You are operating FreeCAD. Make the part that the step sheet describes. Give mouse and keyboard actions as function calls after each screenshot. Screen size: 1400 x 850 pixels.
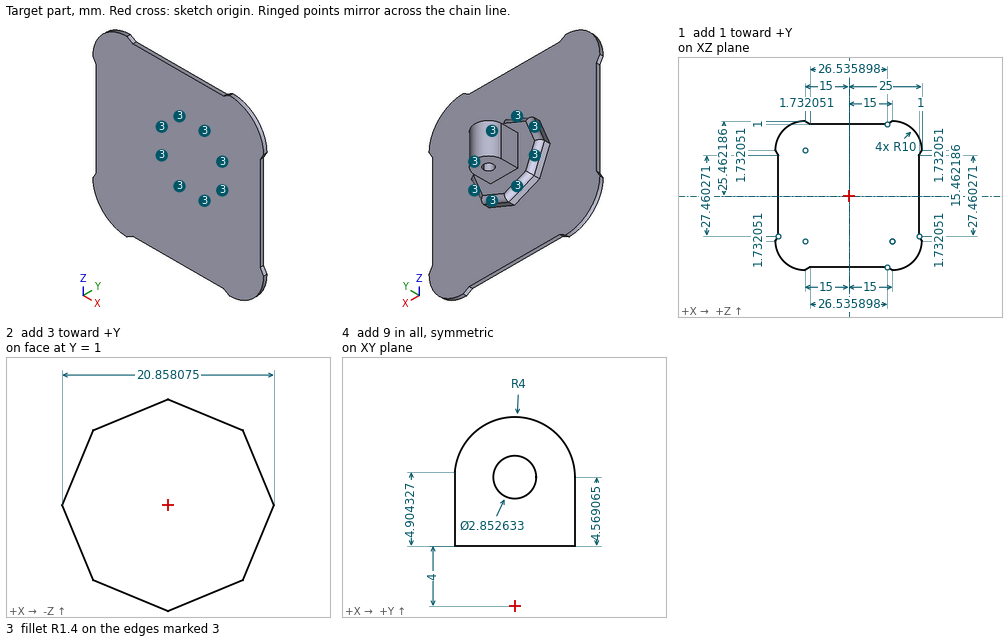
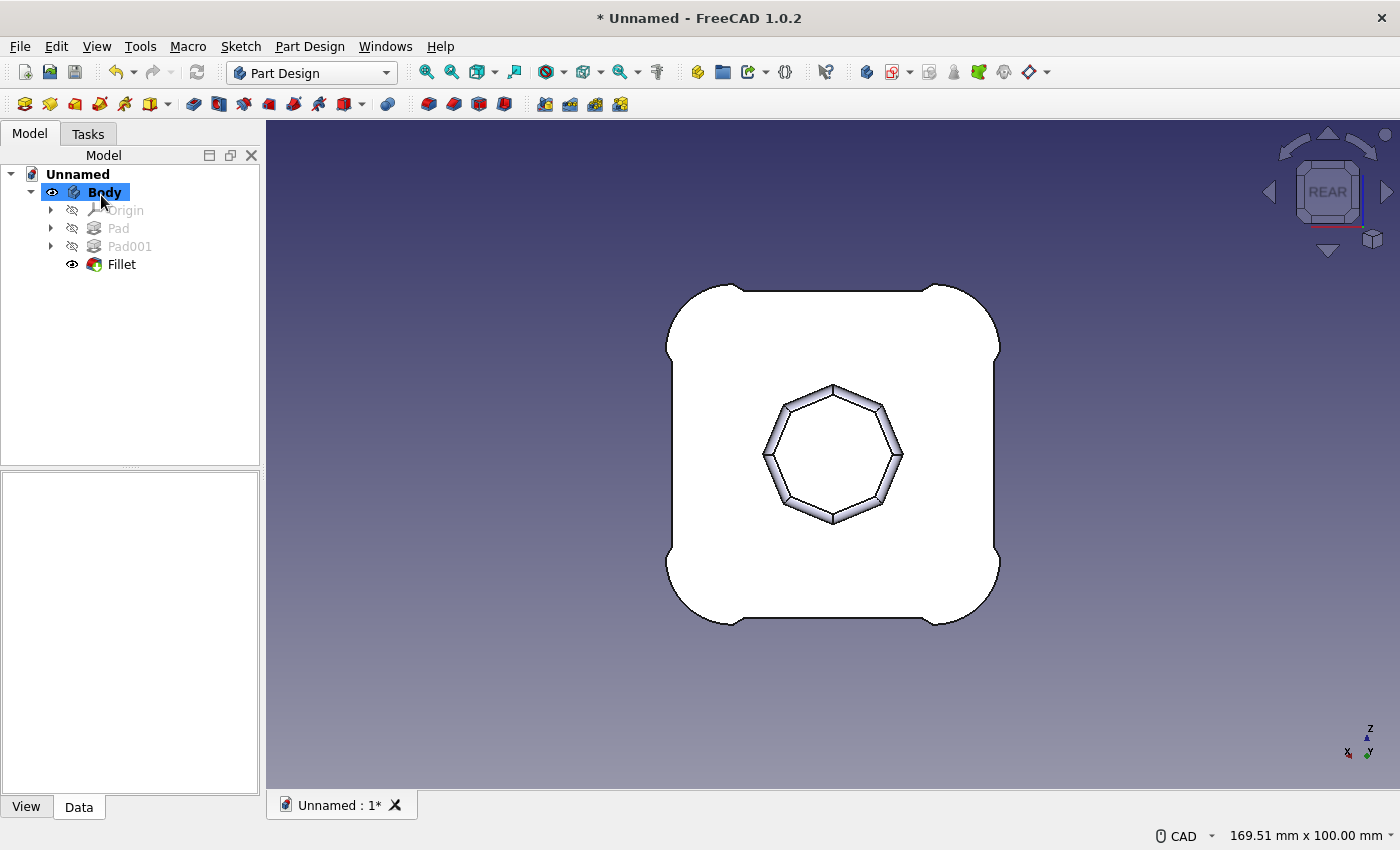
click(892, 72)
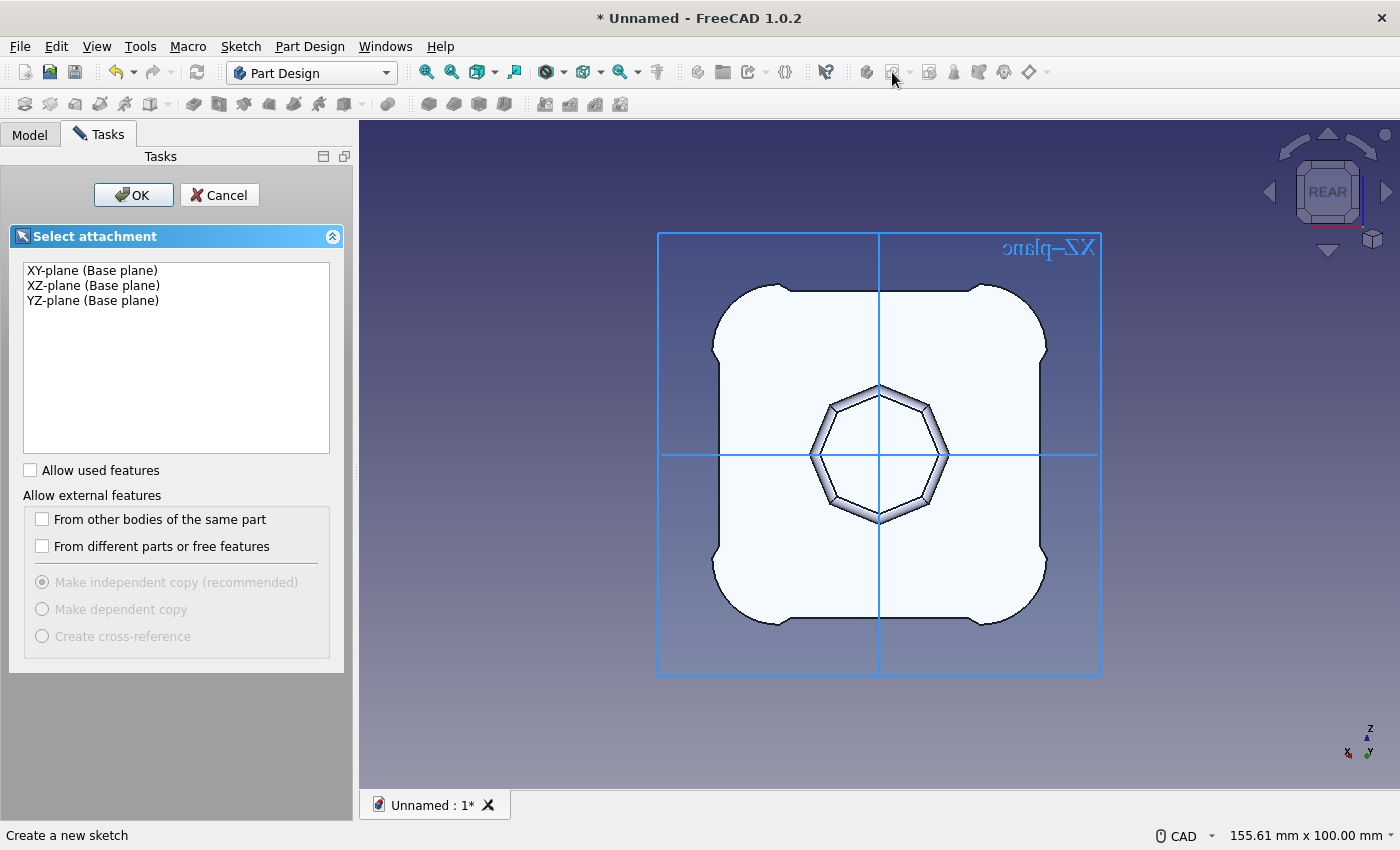
click(84, 270)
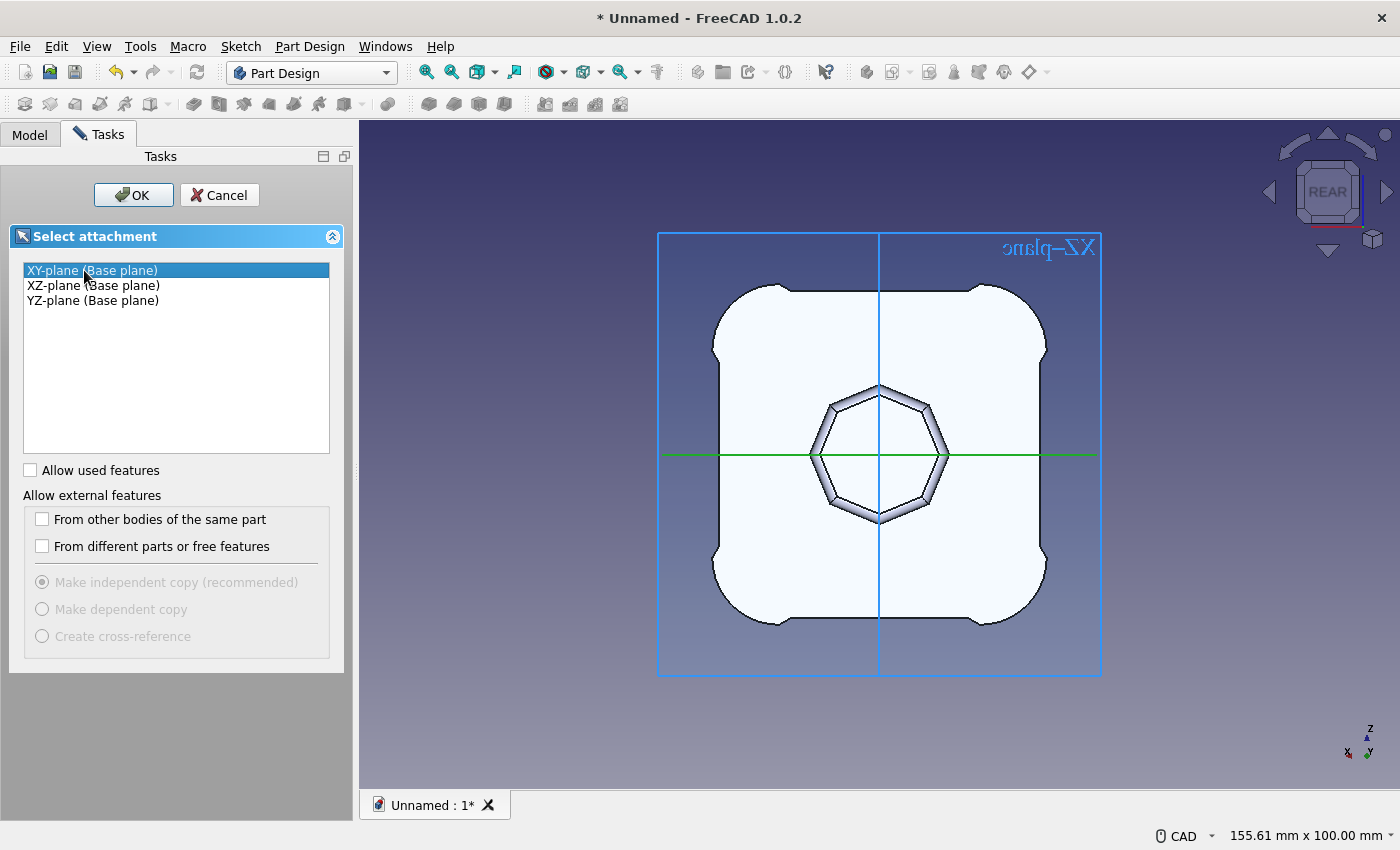
click(134, 195)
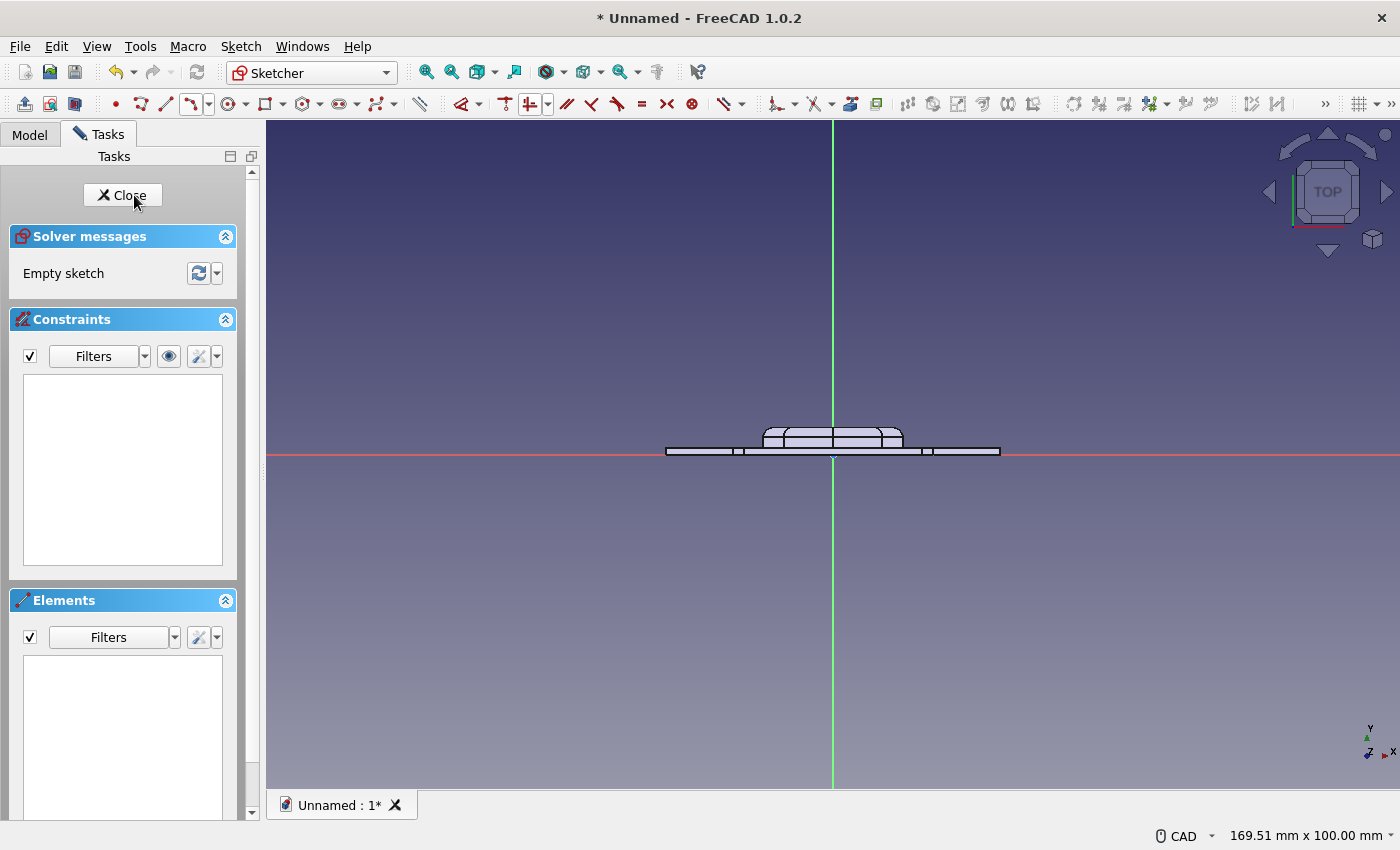
click(75, 104)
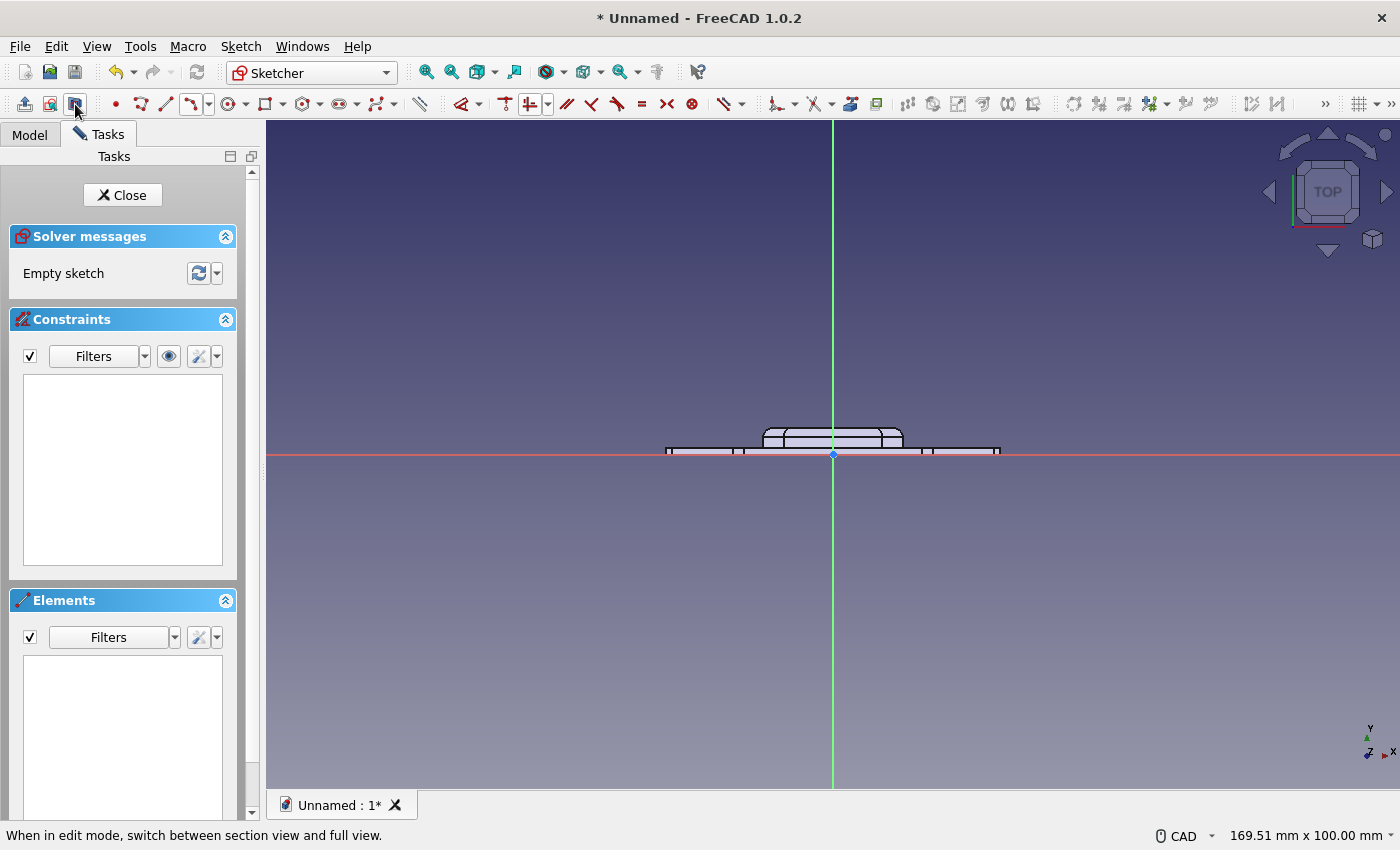
scroll(850, 402, up, 8)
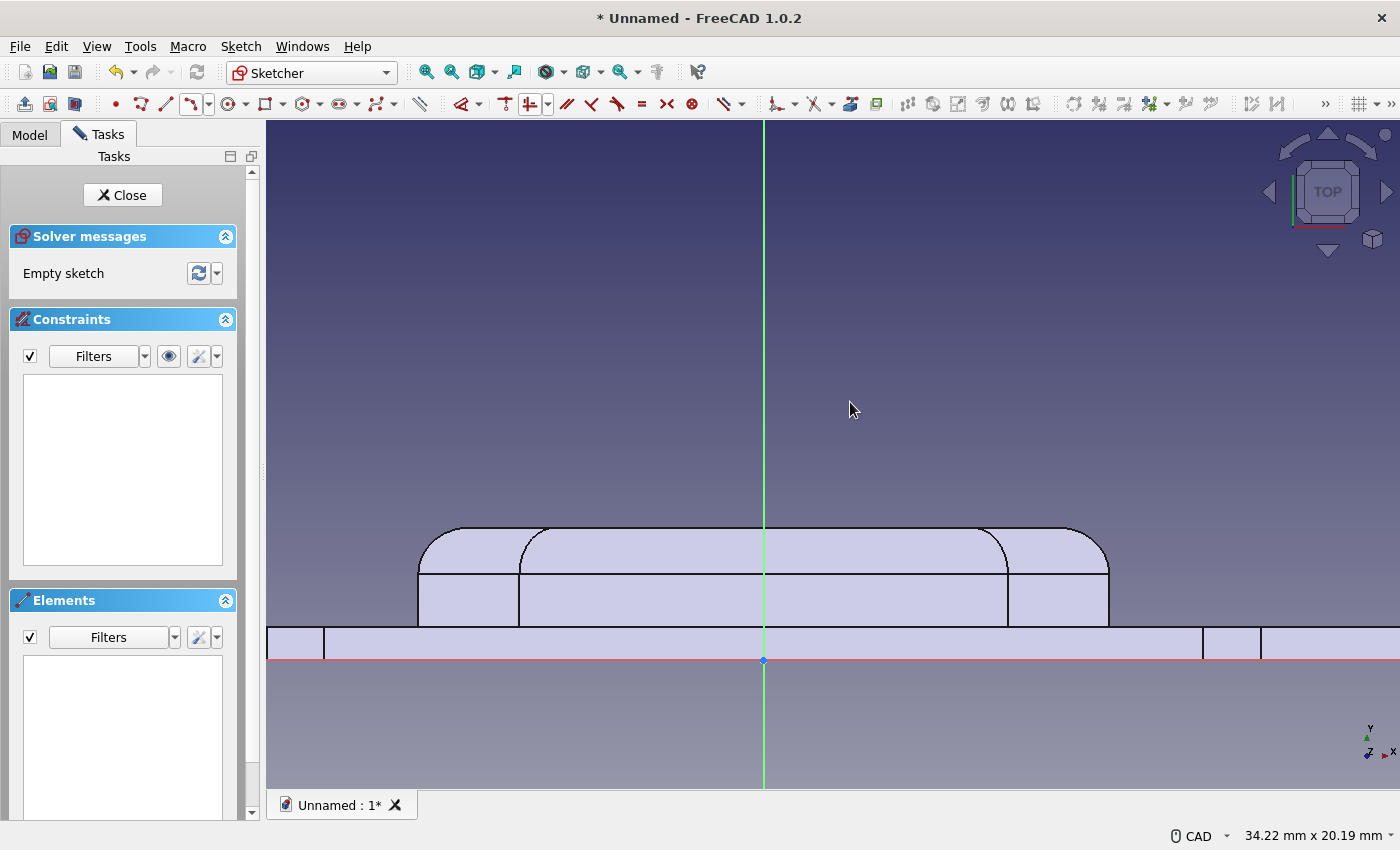
click(141, 104)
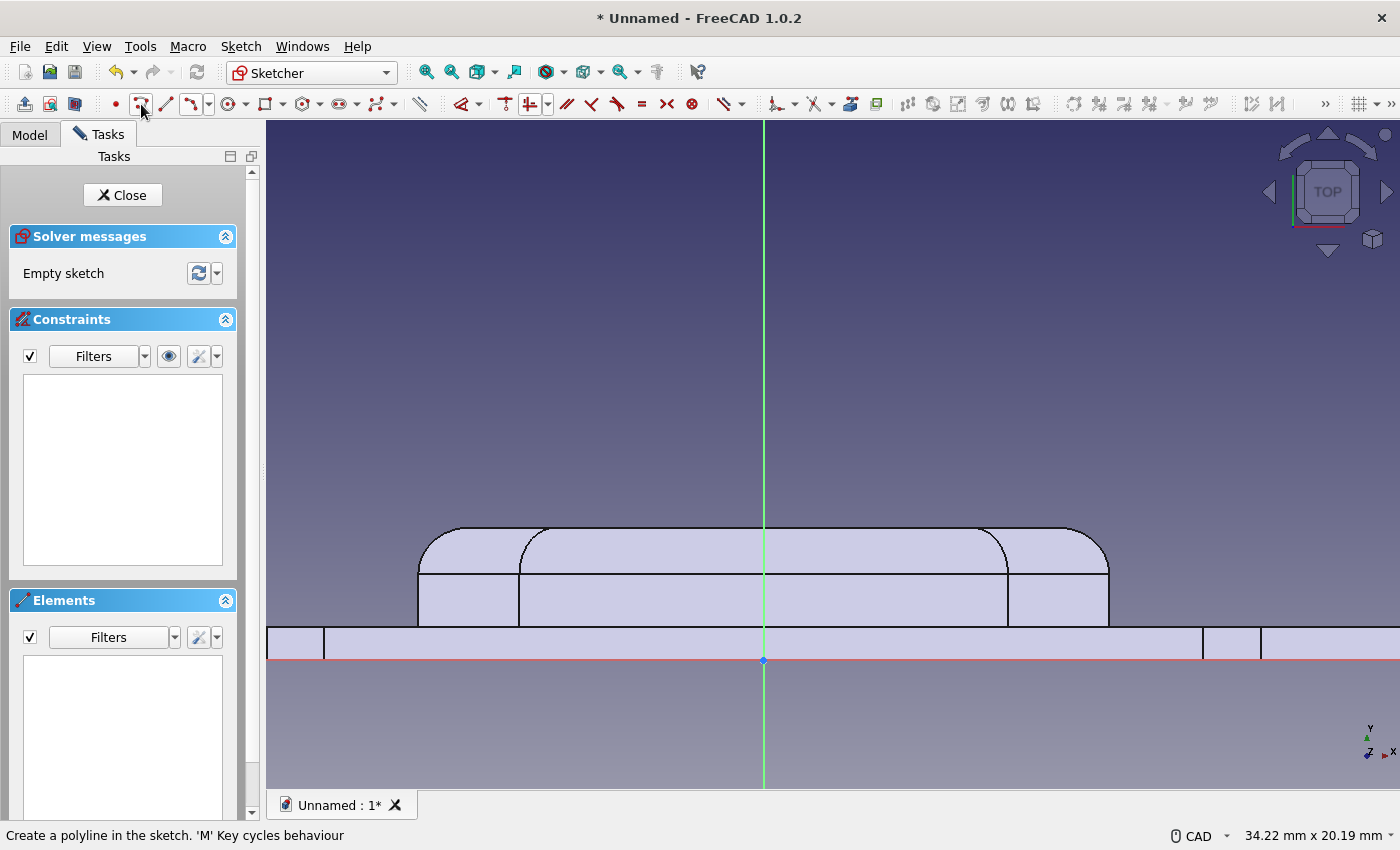
click(632, 365)
click(632, 528)
click(896, 528)
click(896, 376)
right_click(896, 376)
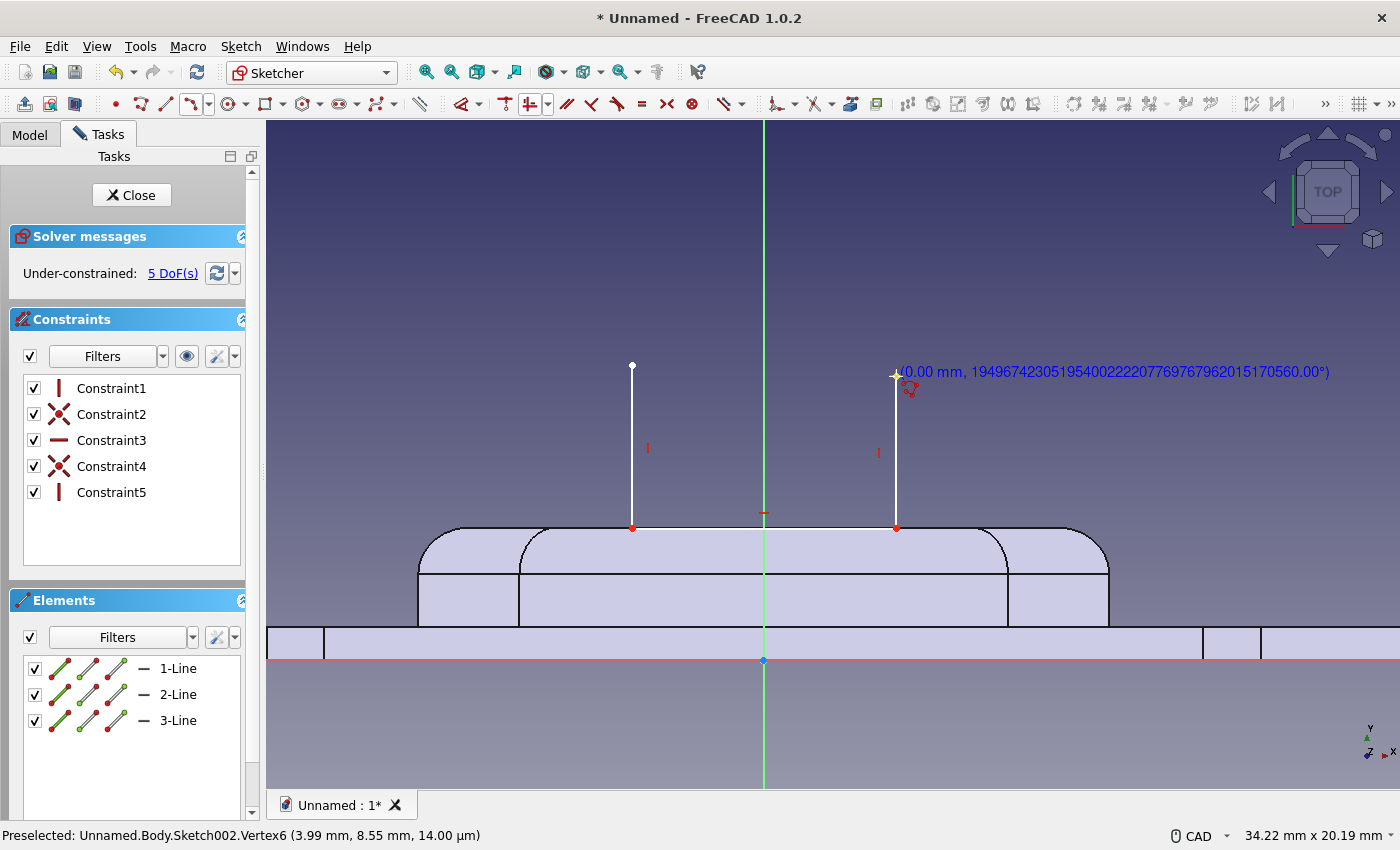
click(190, 104)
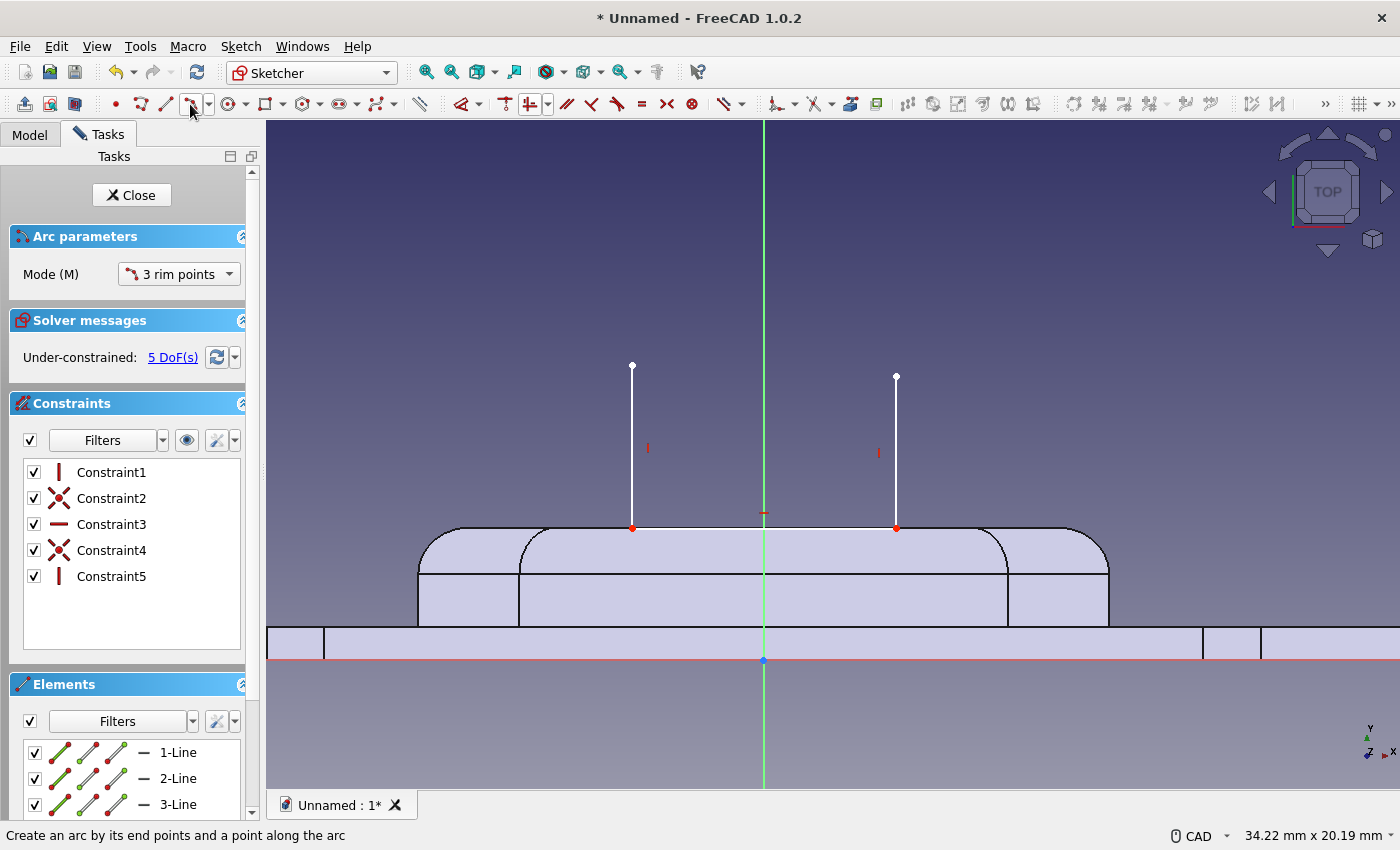
click(896, 377)
click(632, 366)
click(809, 252)